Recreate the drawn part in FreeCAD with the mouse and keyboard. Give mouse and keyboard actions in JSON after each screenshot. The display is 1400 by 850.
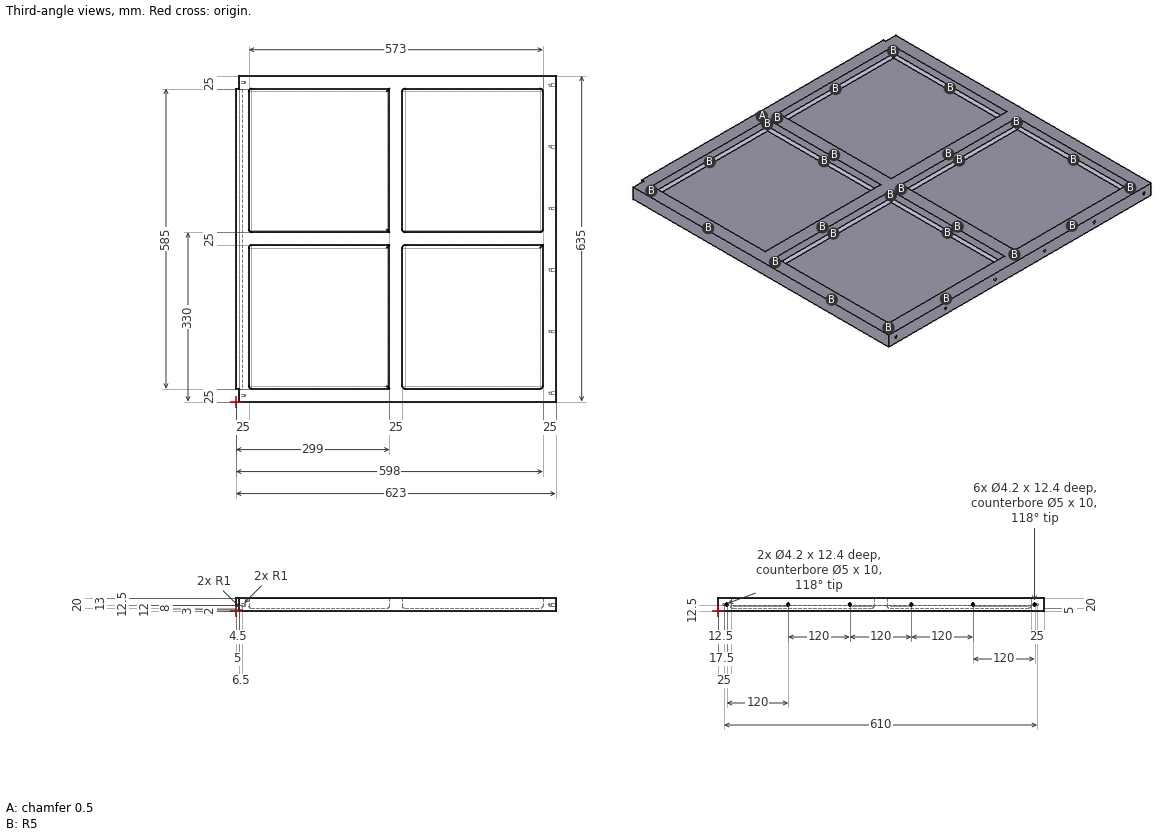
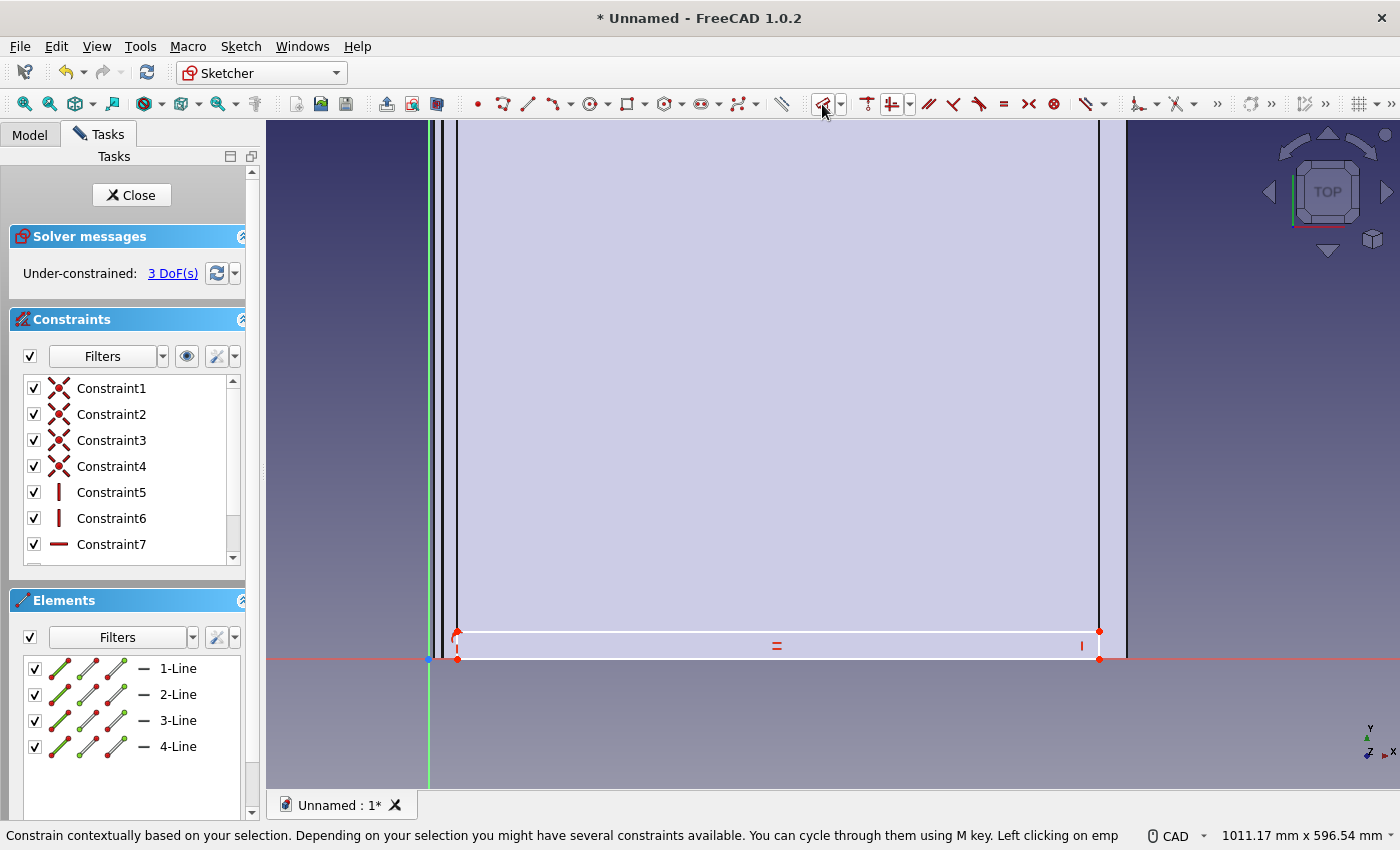
{"action": "scroll", "coordinate": [457, 643], "scroll_direction": "up", "scroll_amount": 2}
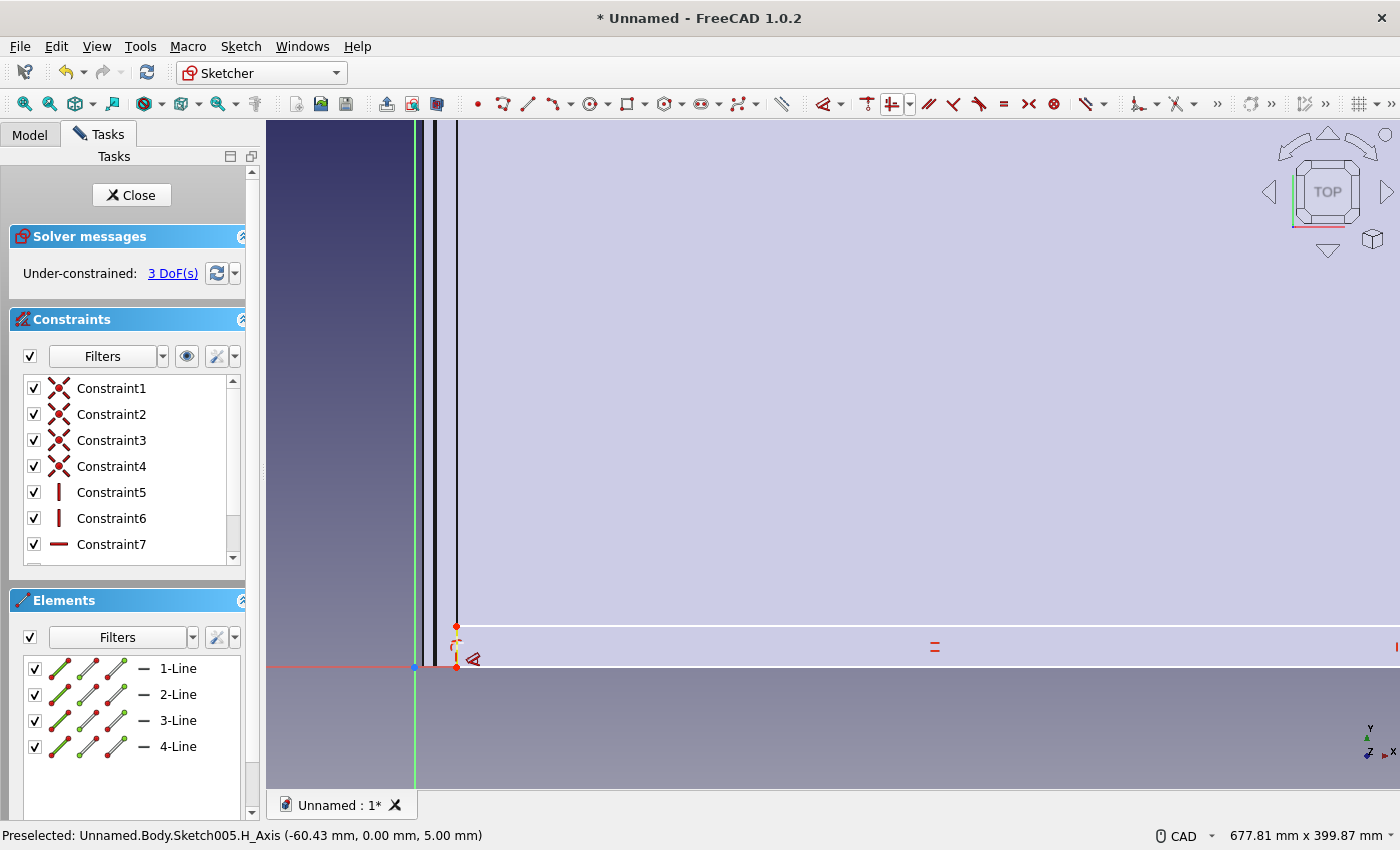
{"action": "left_click", "coordinate": [457, 643]}
{"action": "left_click", "coordinate": [491, 647]}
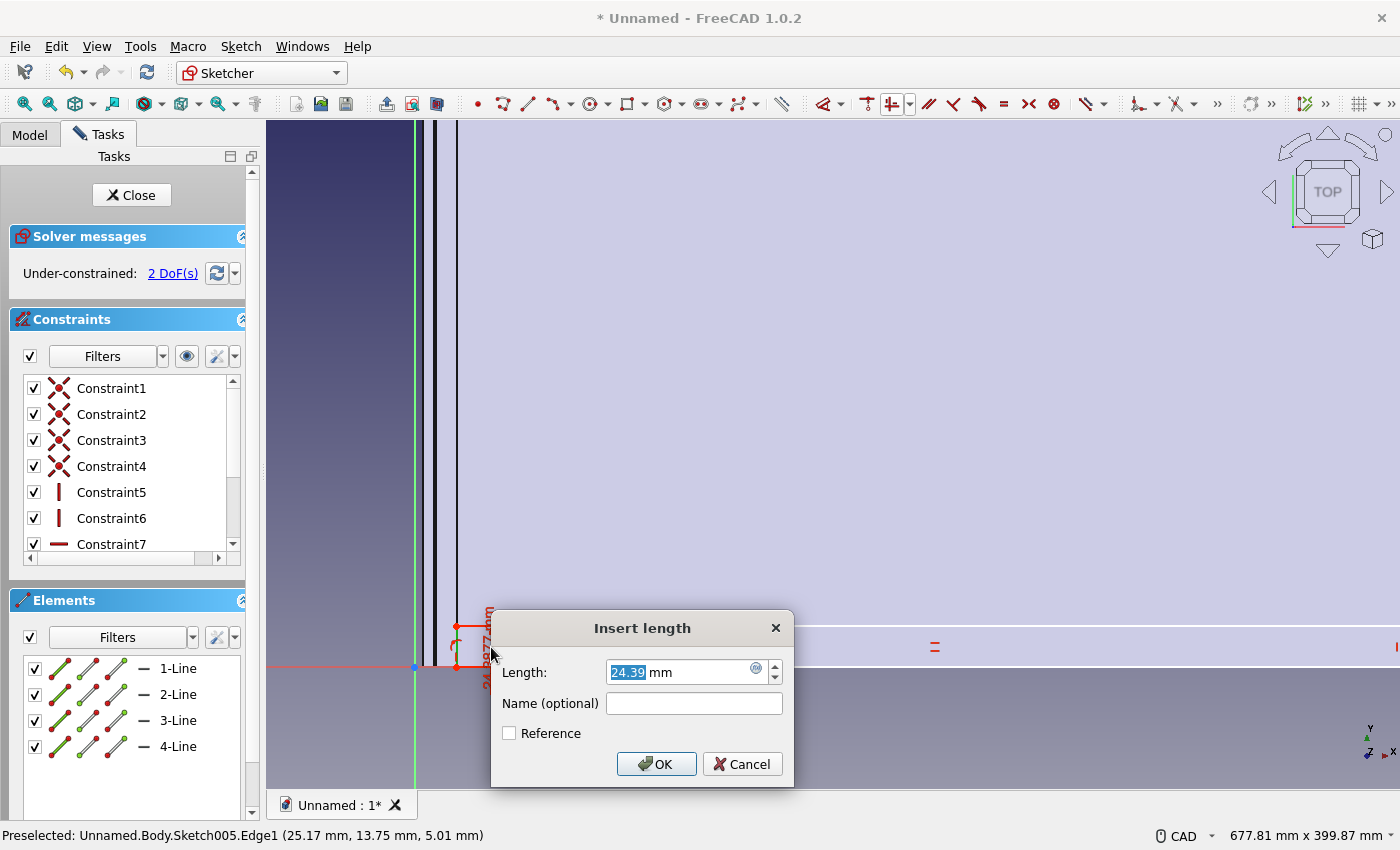
{"action": "type", "text": "25"}
{"action": "key", "text": "Return"}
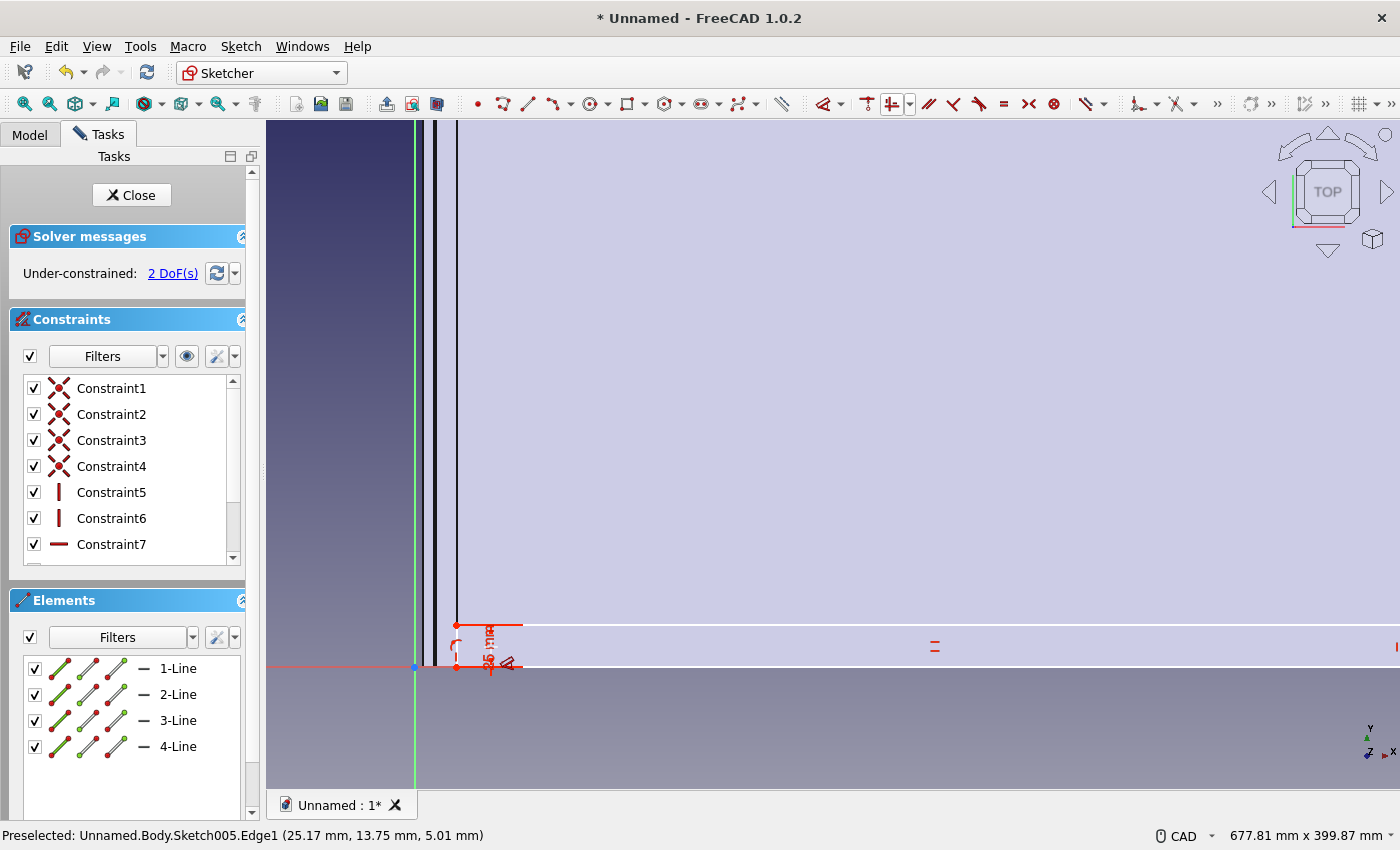
{"action": "left_click", "coordinate": [744, 667]}
{"action": "left_click", "coordinate": [846, 701]}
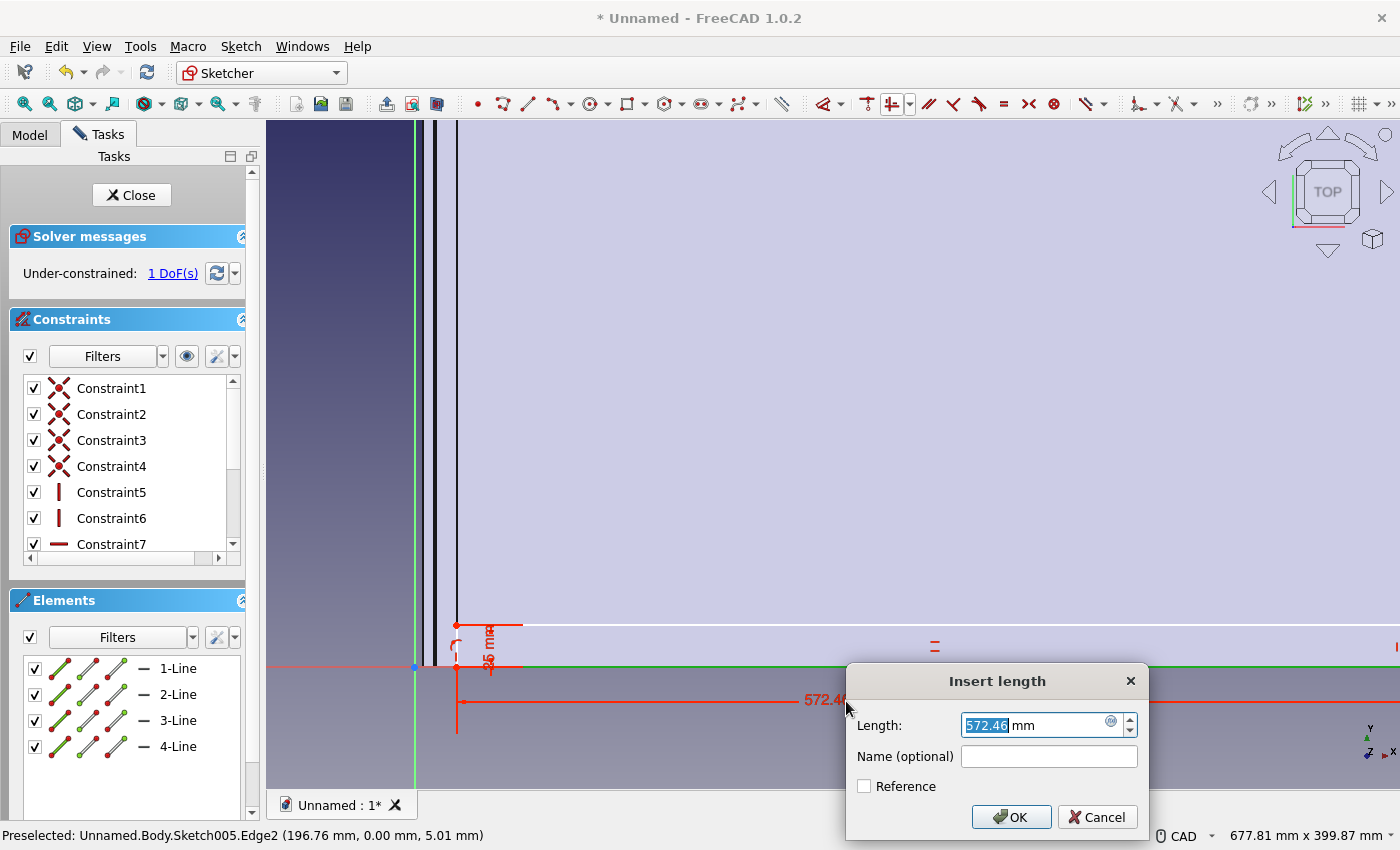
{"action": "type", "text": "573"}
{"action": "key", "text": "Return"}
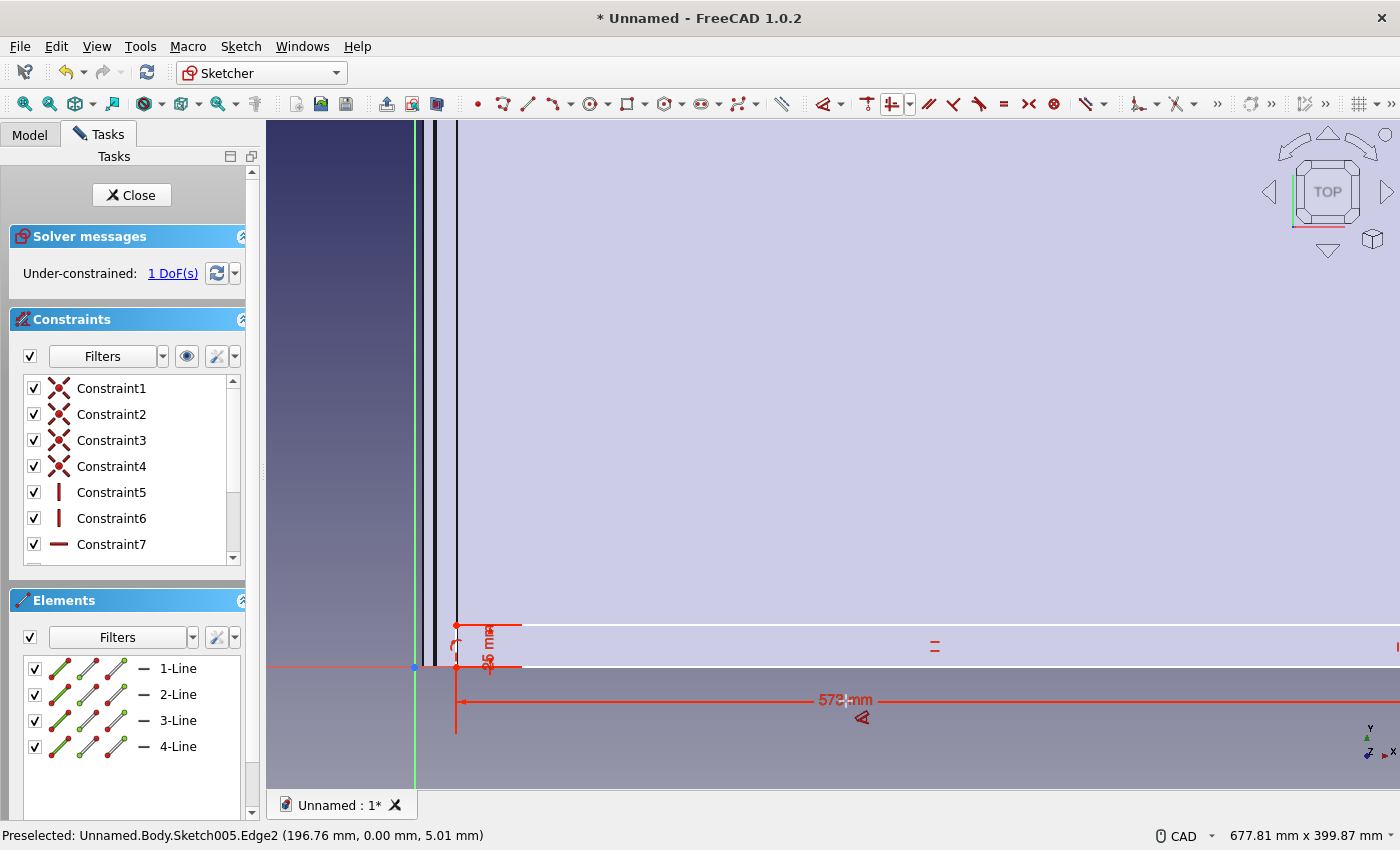
{"action": "left_click", "coordinate": [456, 625]}
{"action": "left_click", "coordinate": [436, 701]}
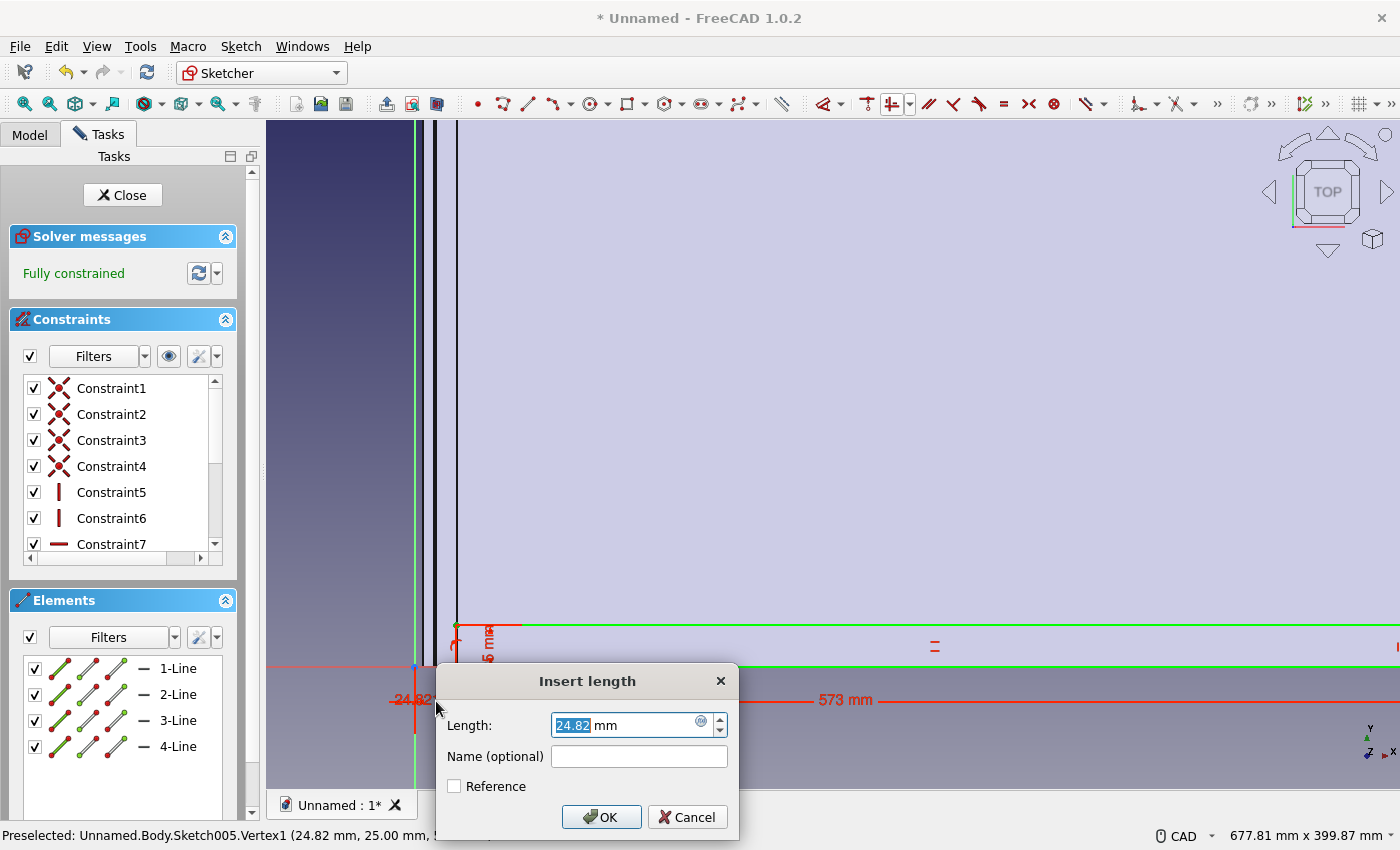
{"action": "type", "text": "25"}
{"action": "key", "text": "Return"}
{"action": "key", "text": "Escape"}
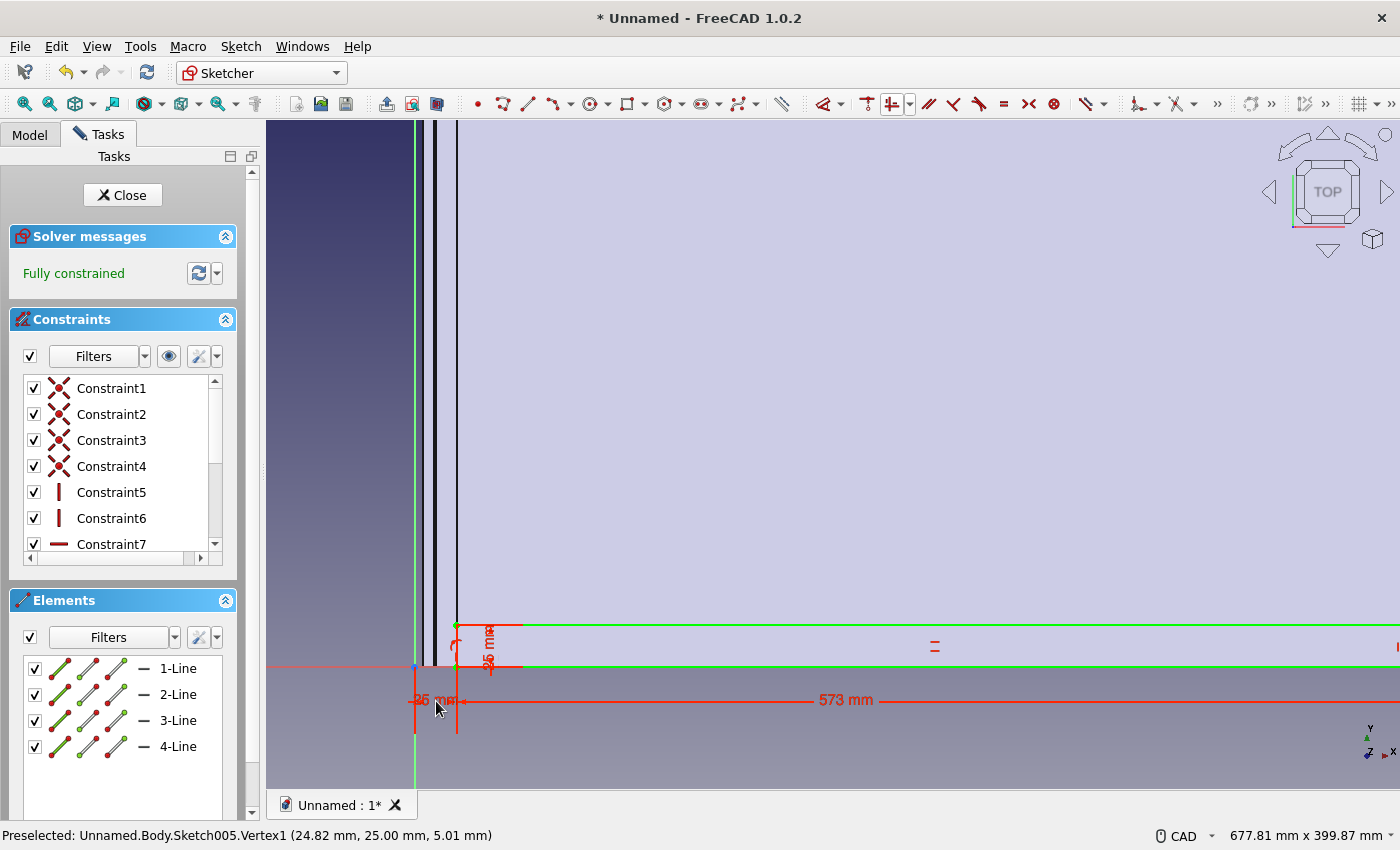
{"action": "left_click", "coordinate": [123, 195]}